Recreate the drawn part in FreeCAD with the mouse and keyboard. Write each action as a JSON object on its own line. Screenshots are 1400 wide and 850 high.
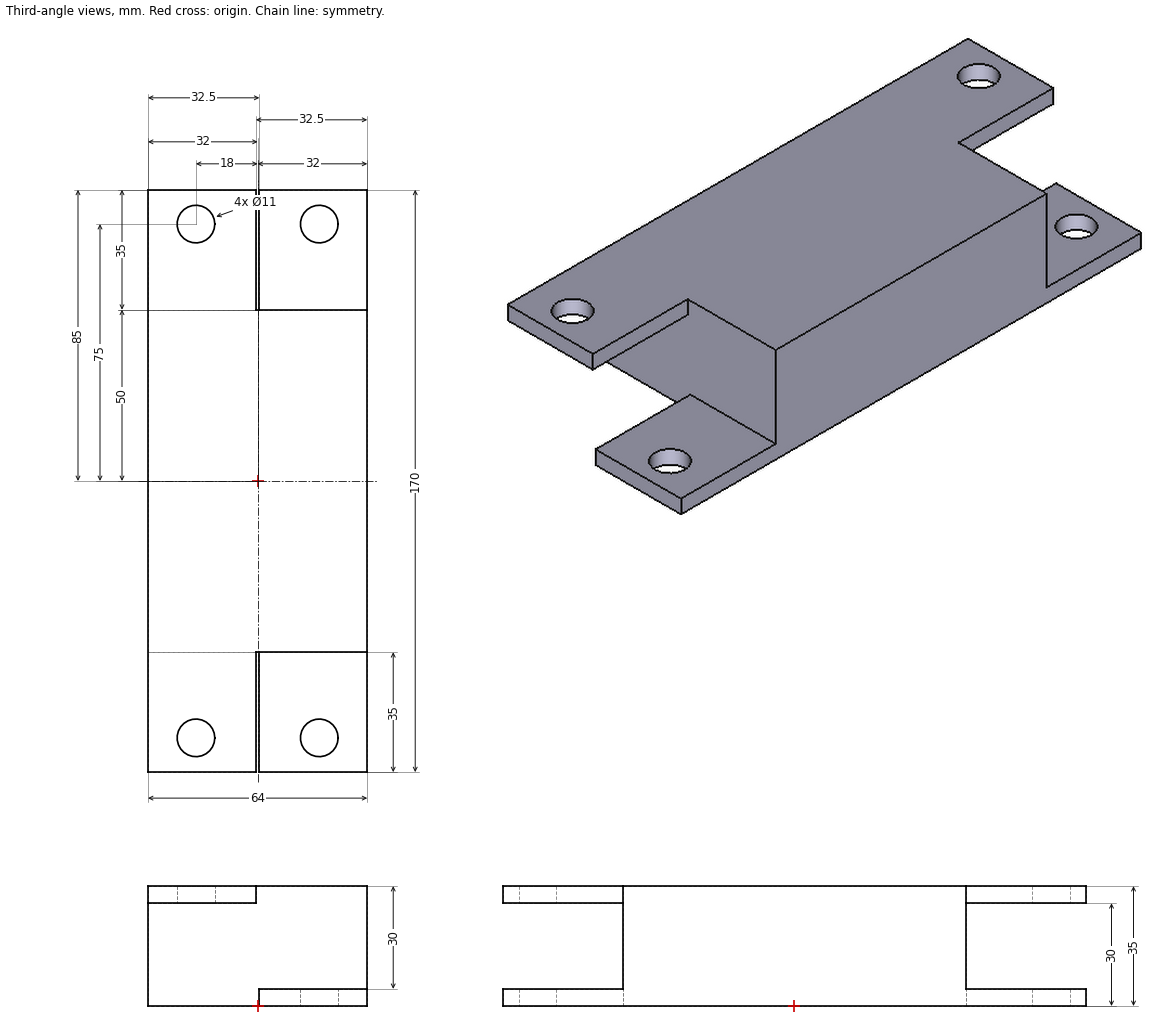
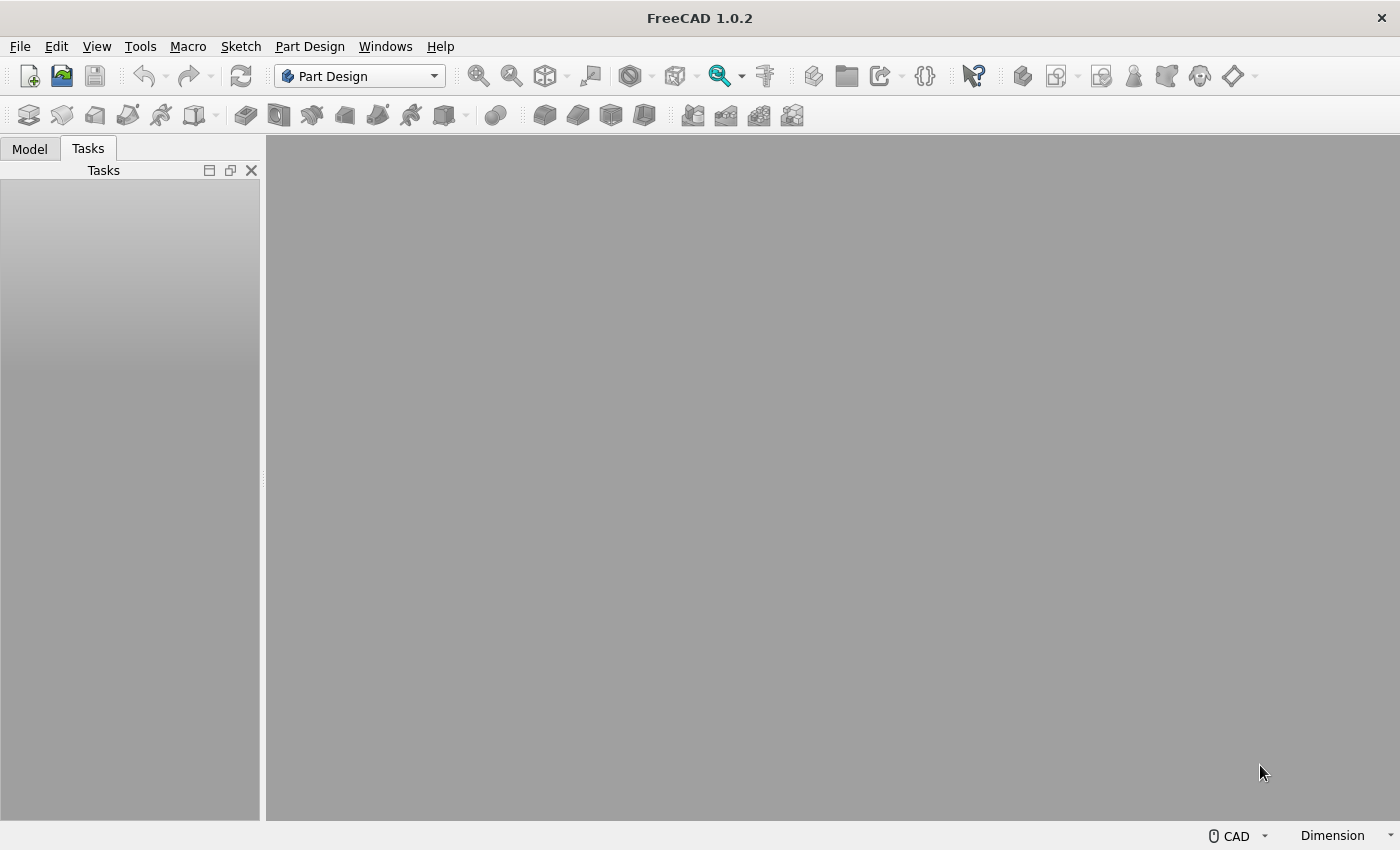
{"action": "left_click", "coordinate": [29, 76]}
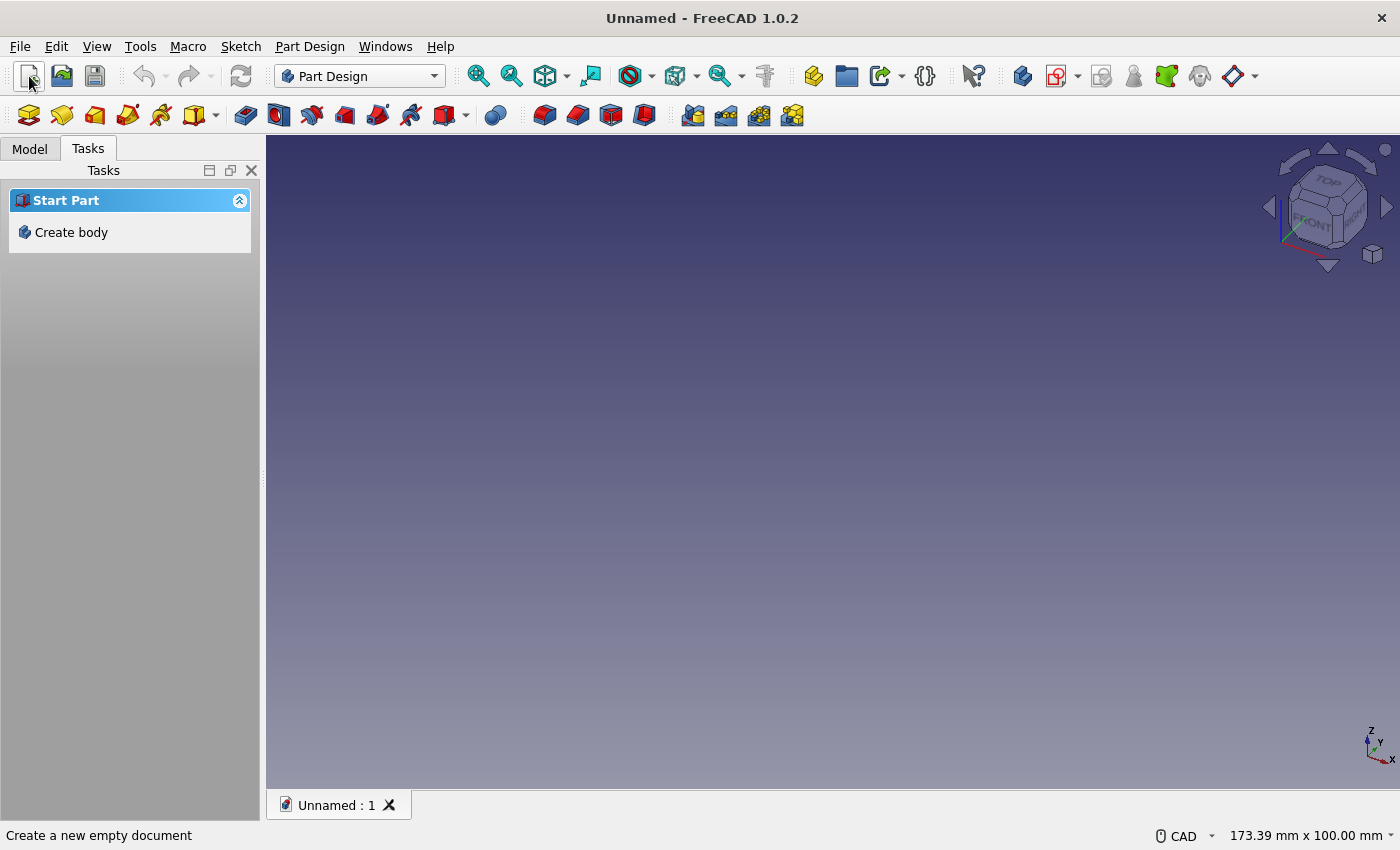
{"action": "left_click", "coordinate": [1056, 76]}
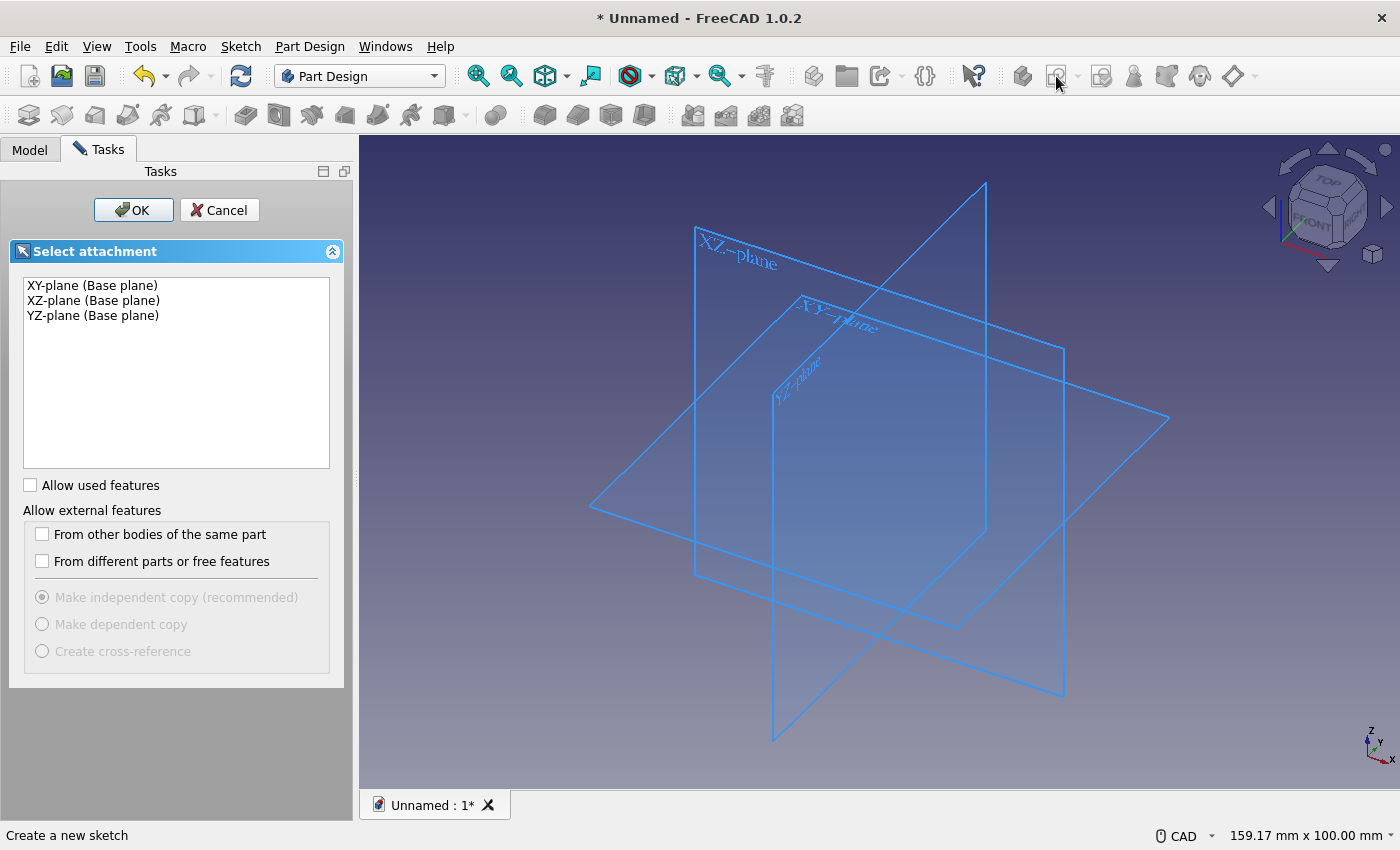
{"action": "left_click", "coordinate": [84, 286]}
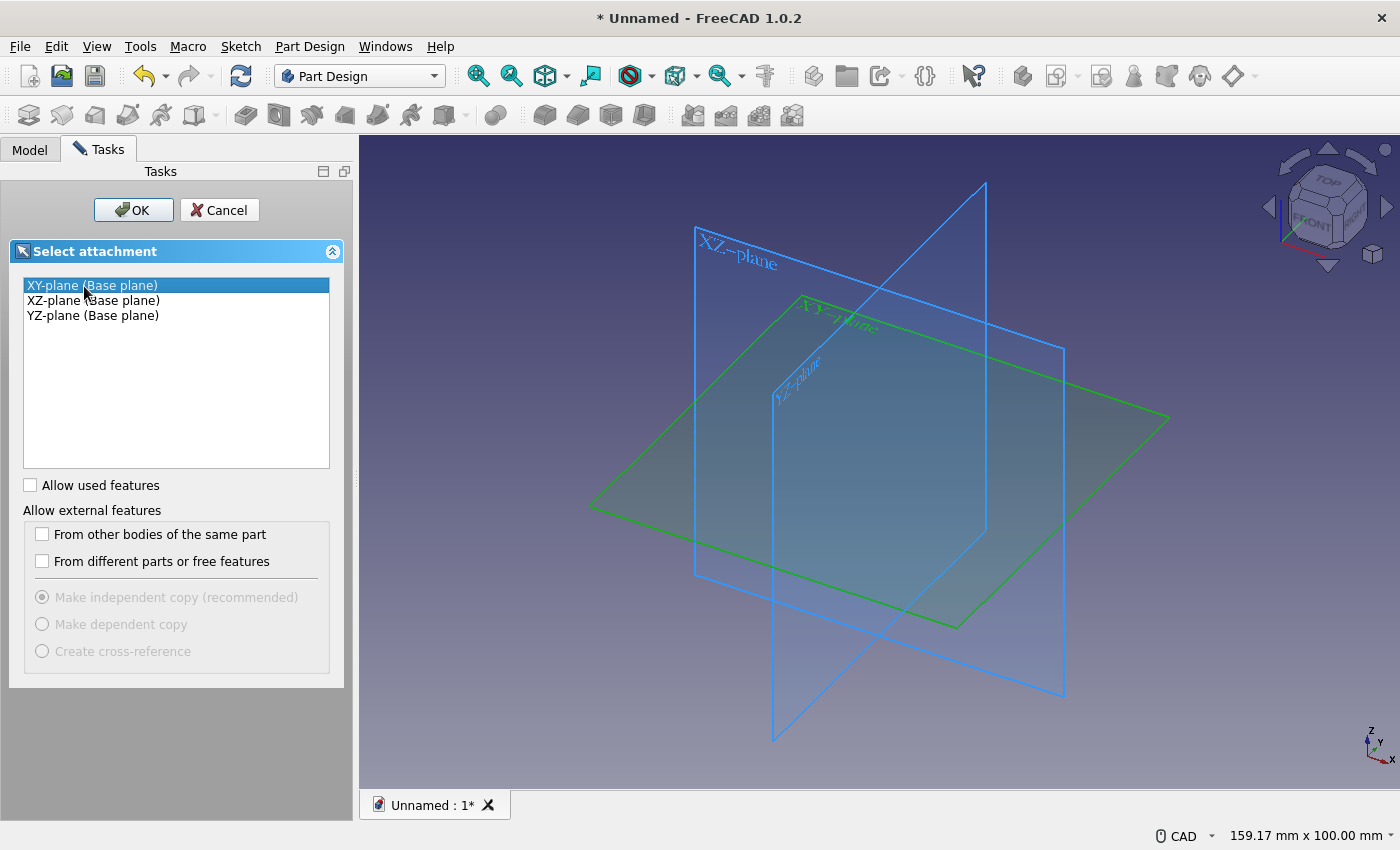
{"action": "left_click", "coordinate": [134, 210]}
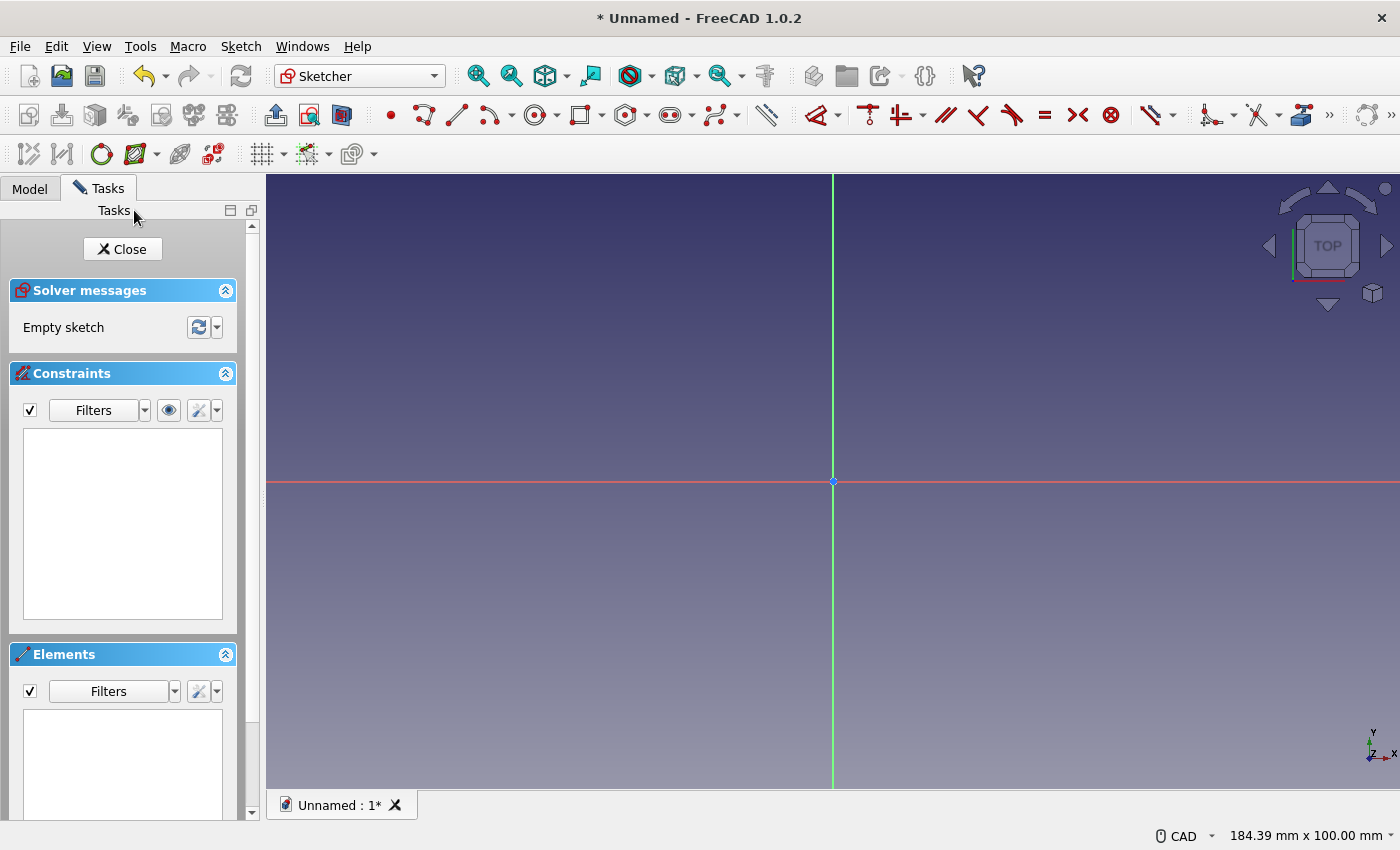
{"action": "scroll", "coordinate": [725, 482], "scroll_direction": "down", "scroll_amount": 5}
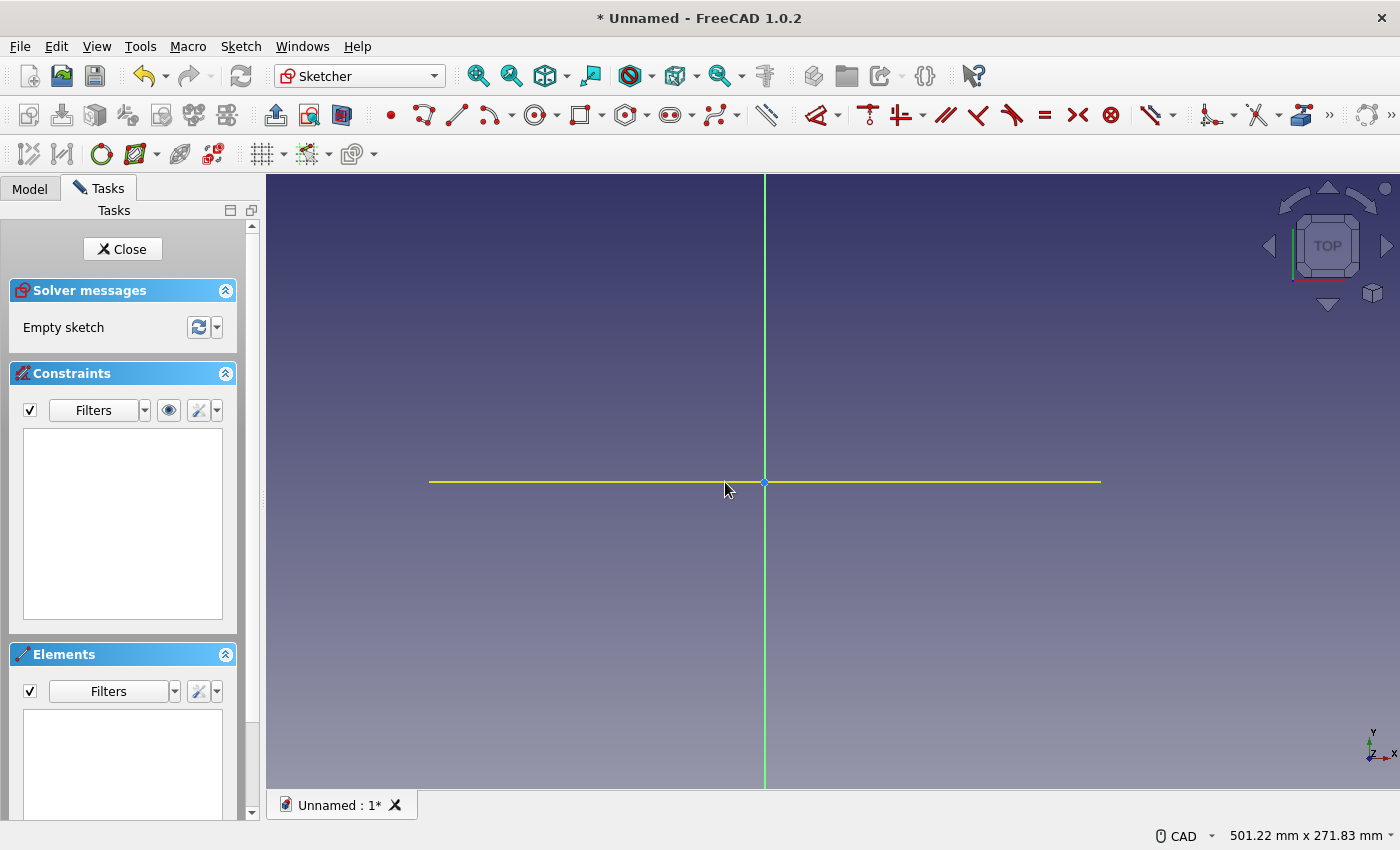
{"action": "left_click", "coordinate": [602, 116]}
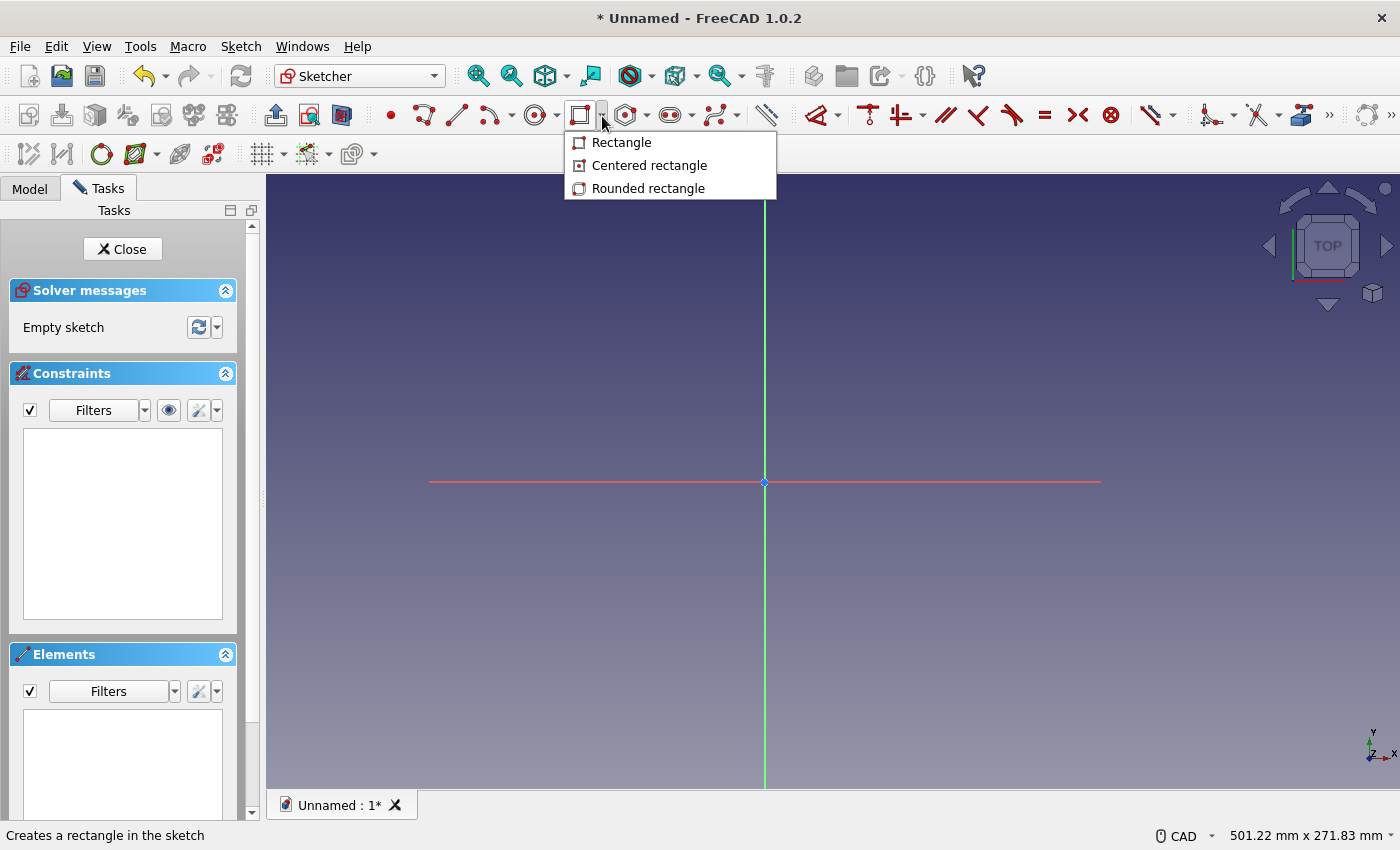
{"action": "left_click", "coordinate": [670, 166]}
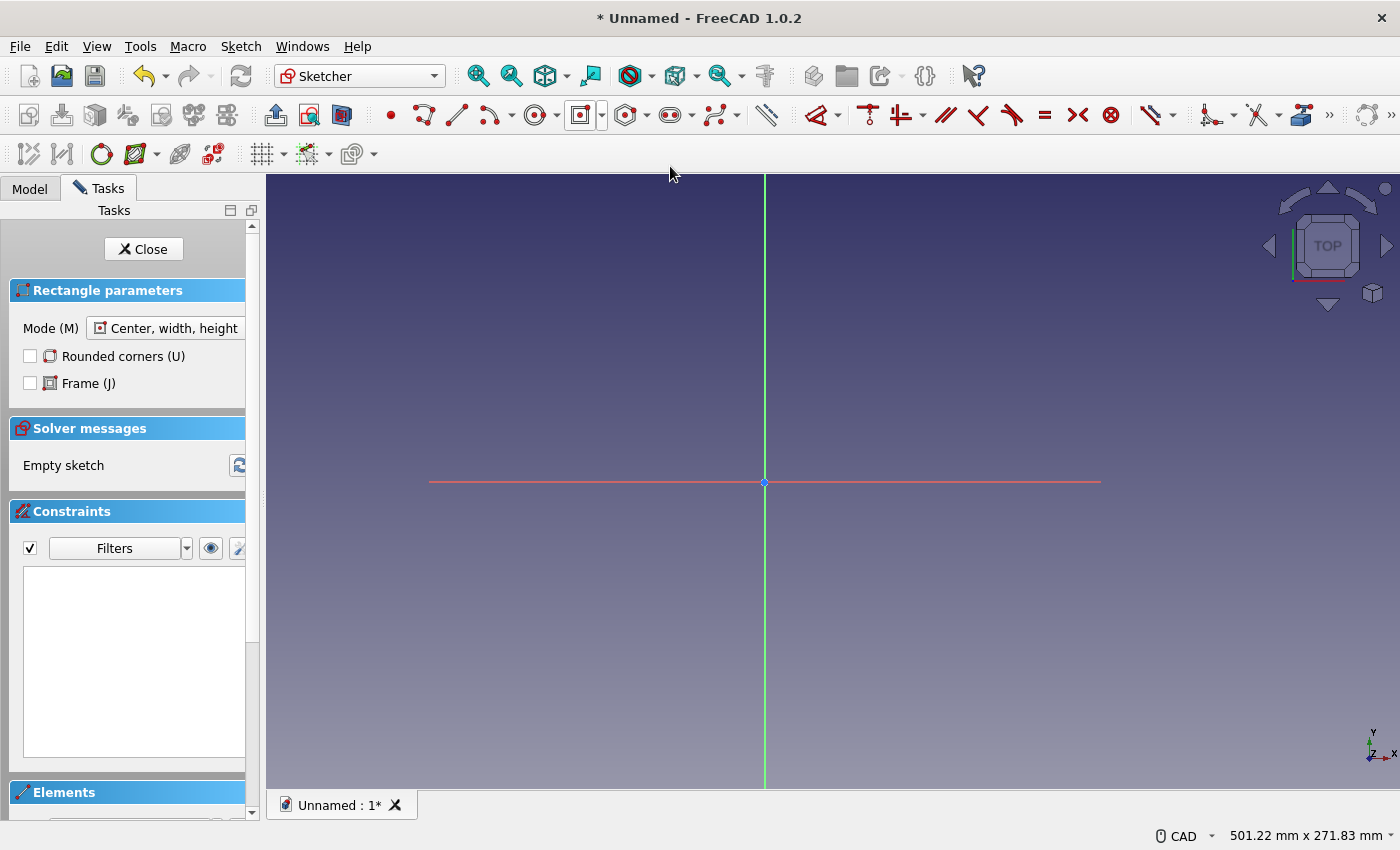
{"action": "left_click", "coordinate": [765, 482]}
{"action": "mouse_move", "coordinate": [837, 290]}